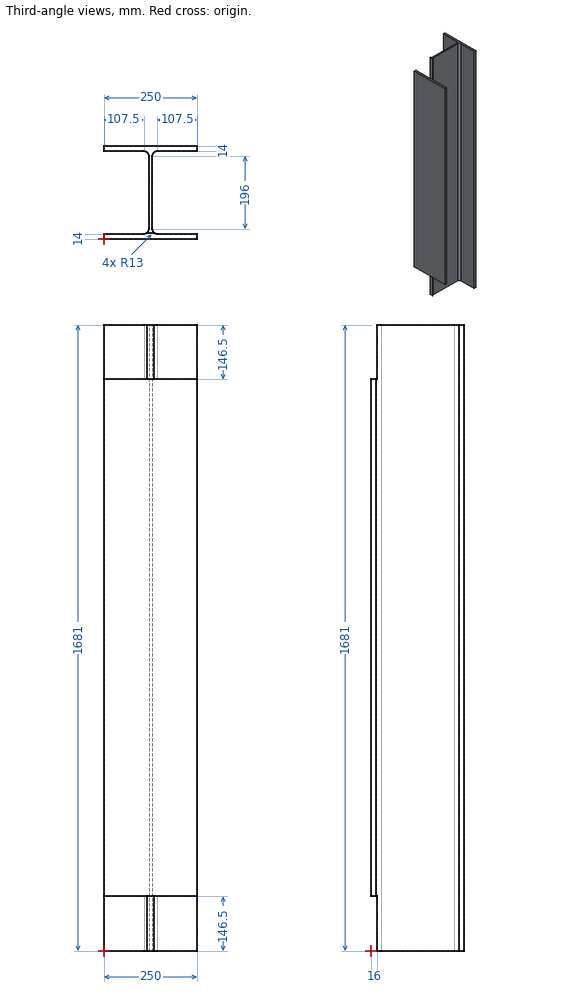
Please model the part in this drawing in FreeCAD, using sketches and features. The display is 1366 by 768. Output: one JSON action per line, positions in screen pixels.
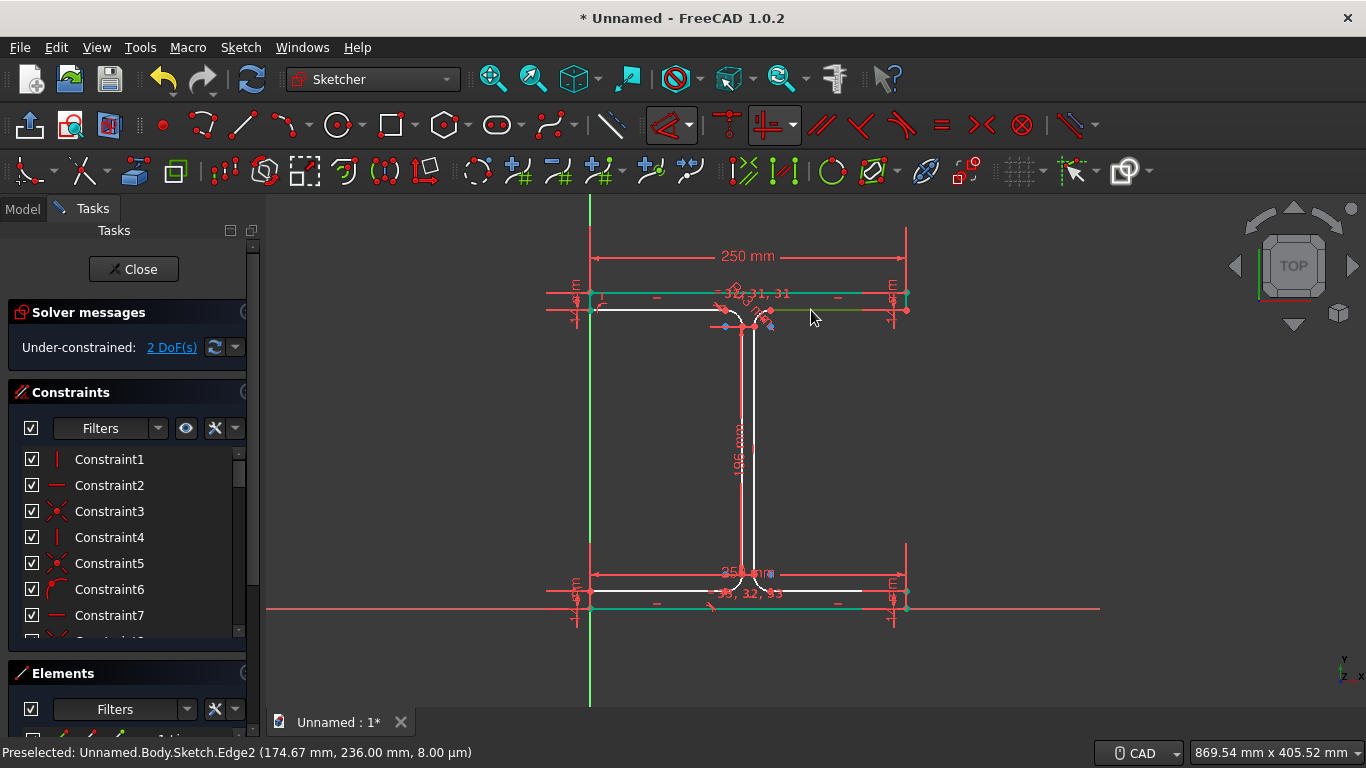
{"action": "left_click", "coordinate": [692, 126]}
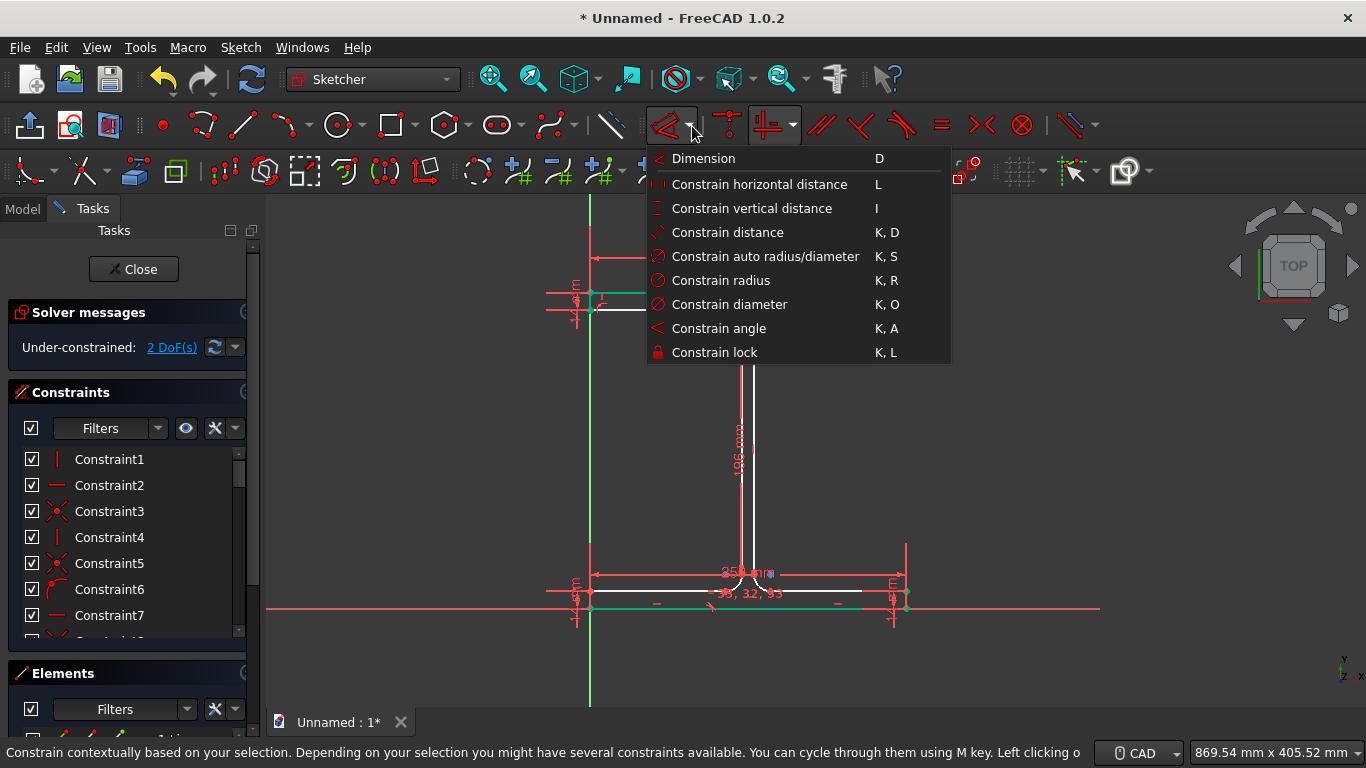
{"action": "left_click", "coordinate": [799, 184]}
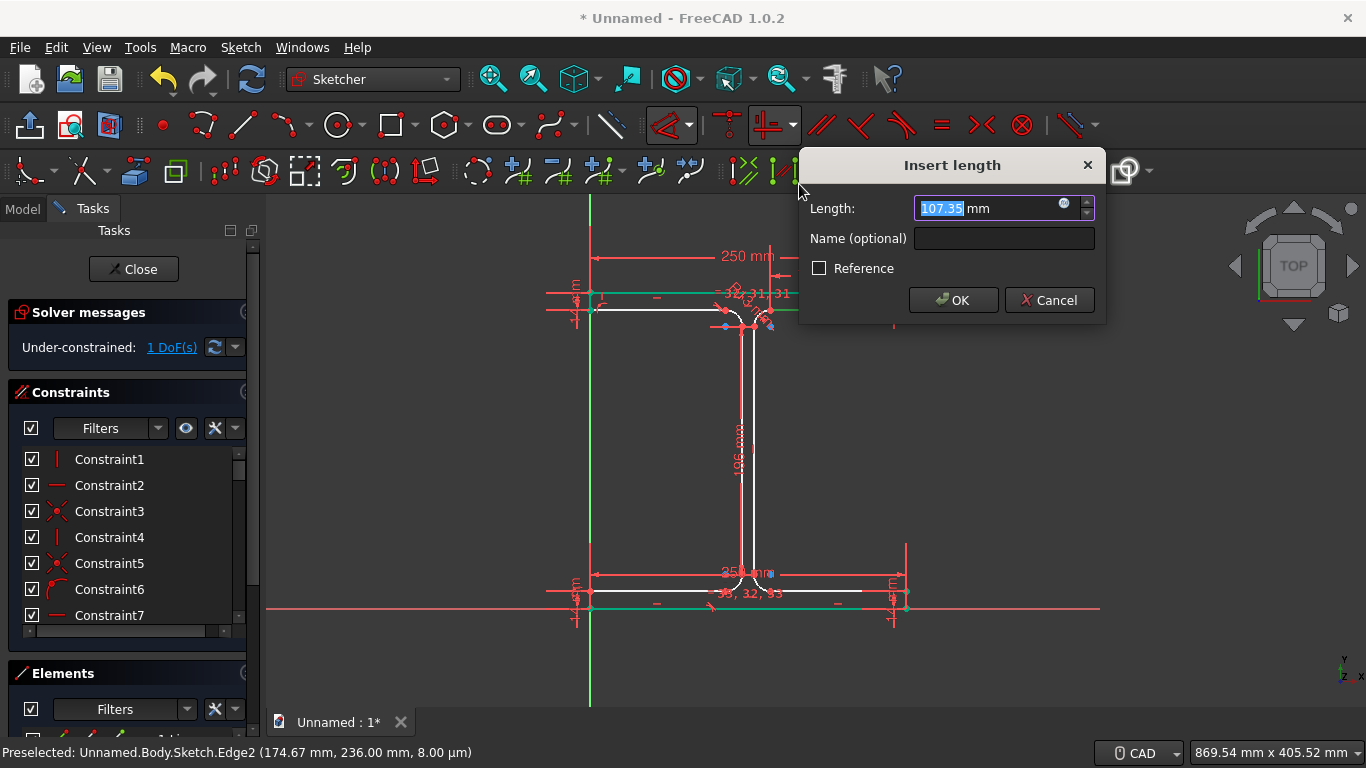
{"action": "type", "text": "107.5"}
{"action": "key", "text": "Return"}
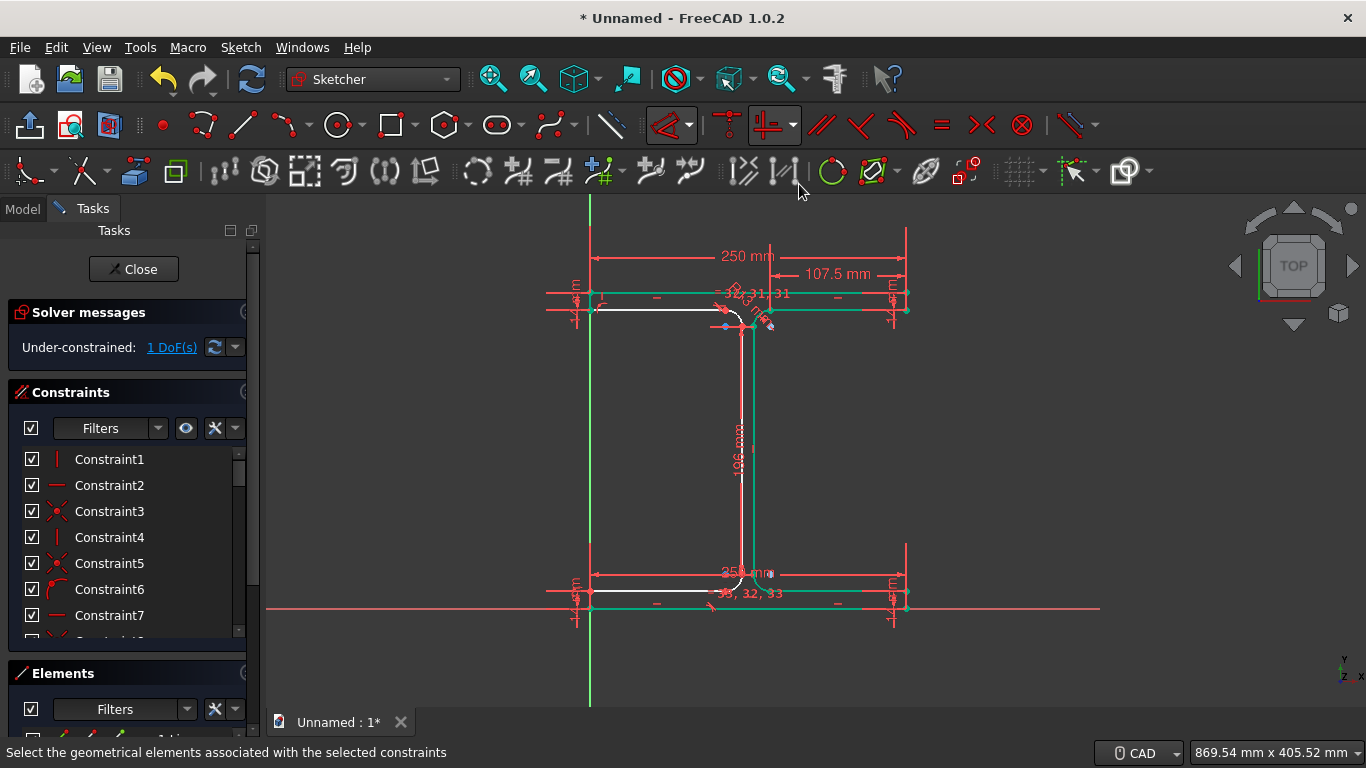
{"action": "left_click", "coordinate": [631, 310]}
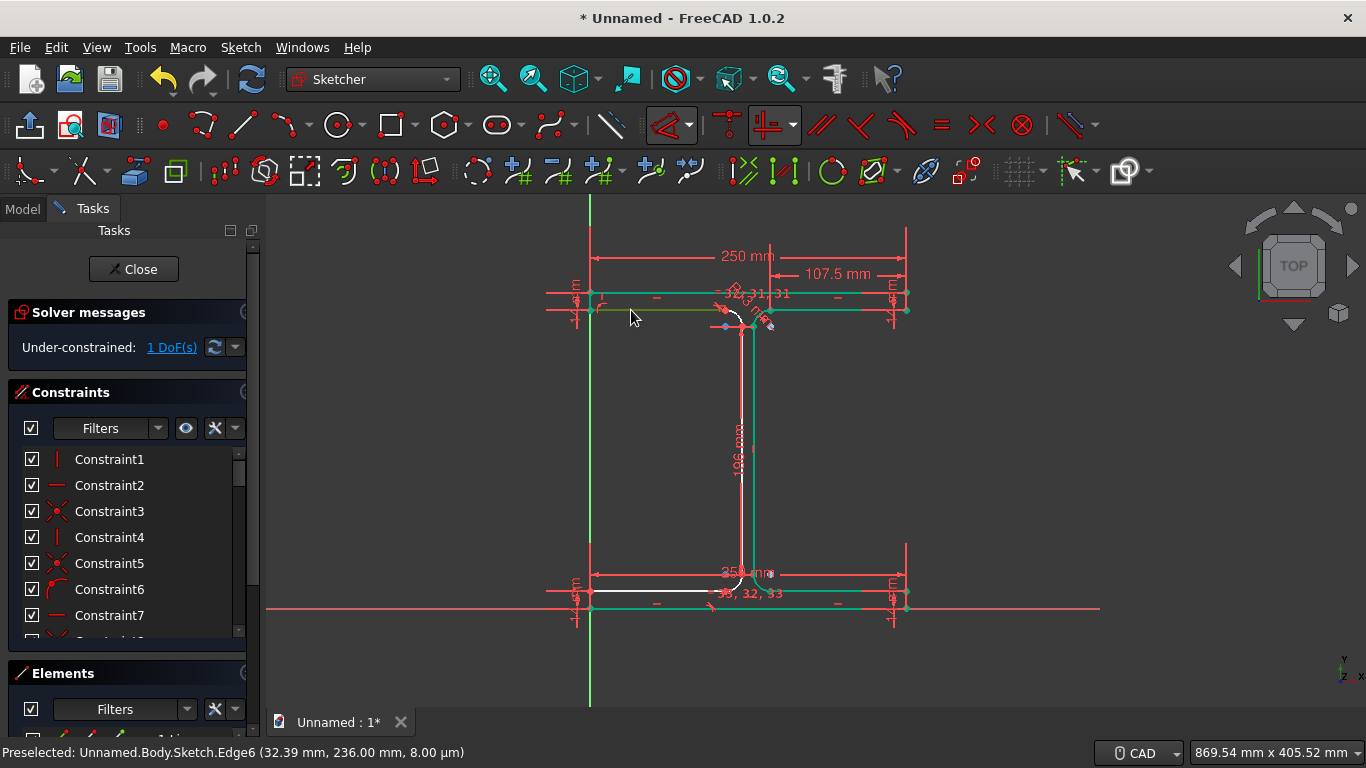
{"action": "left_click", "coordinate": [692, 126]}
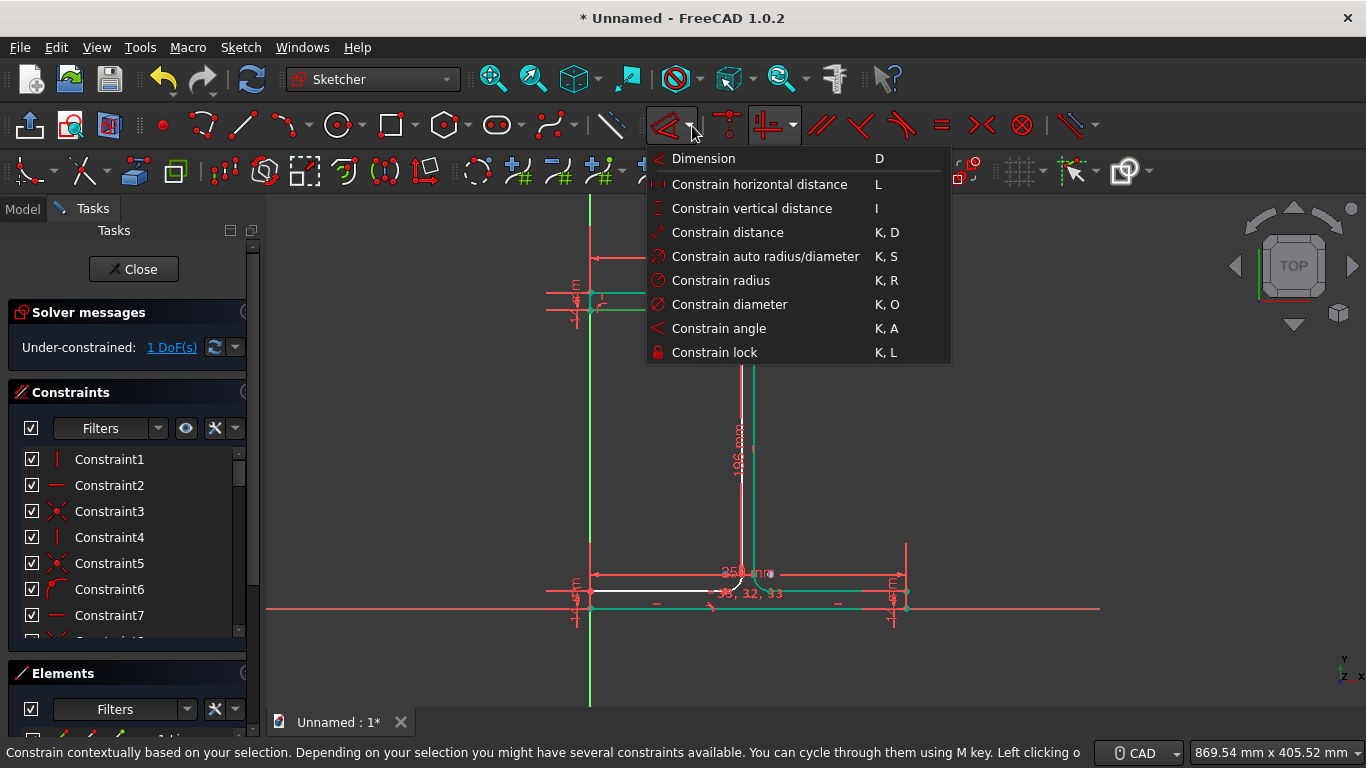
{"action": "left_click", "coordinate": [799, 184]}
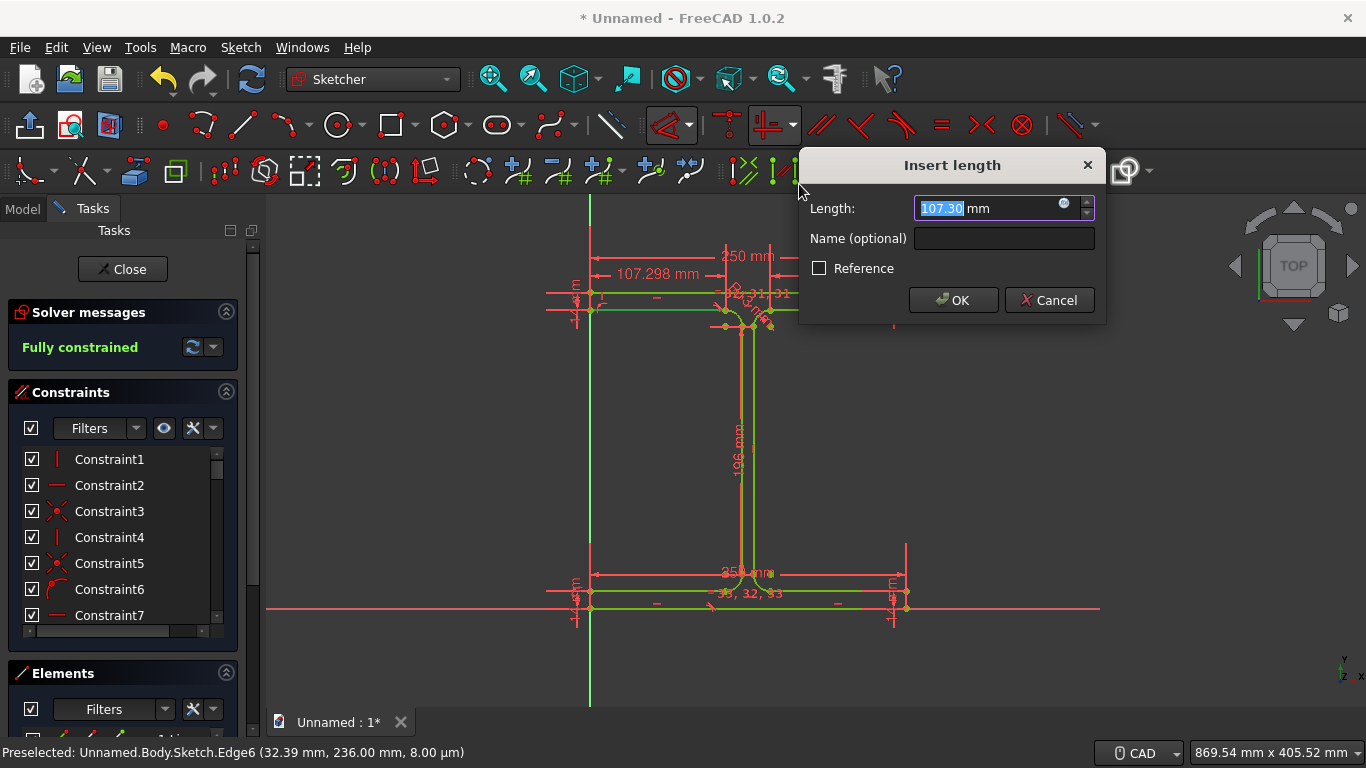
{"action": "type", "text": "107.5"}
{"action": "key", "text": "Return"}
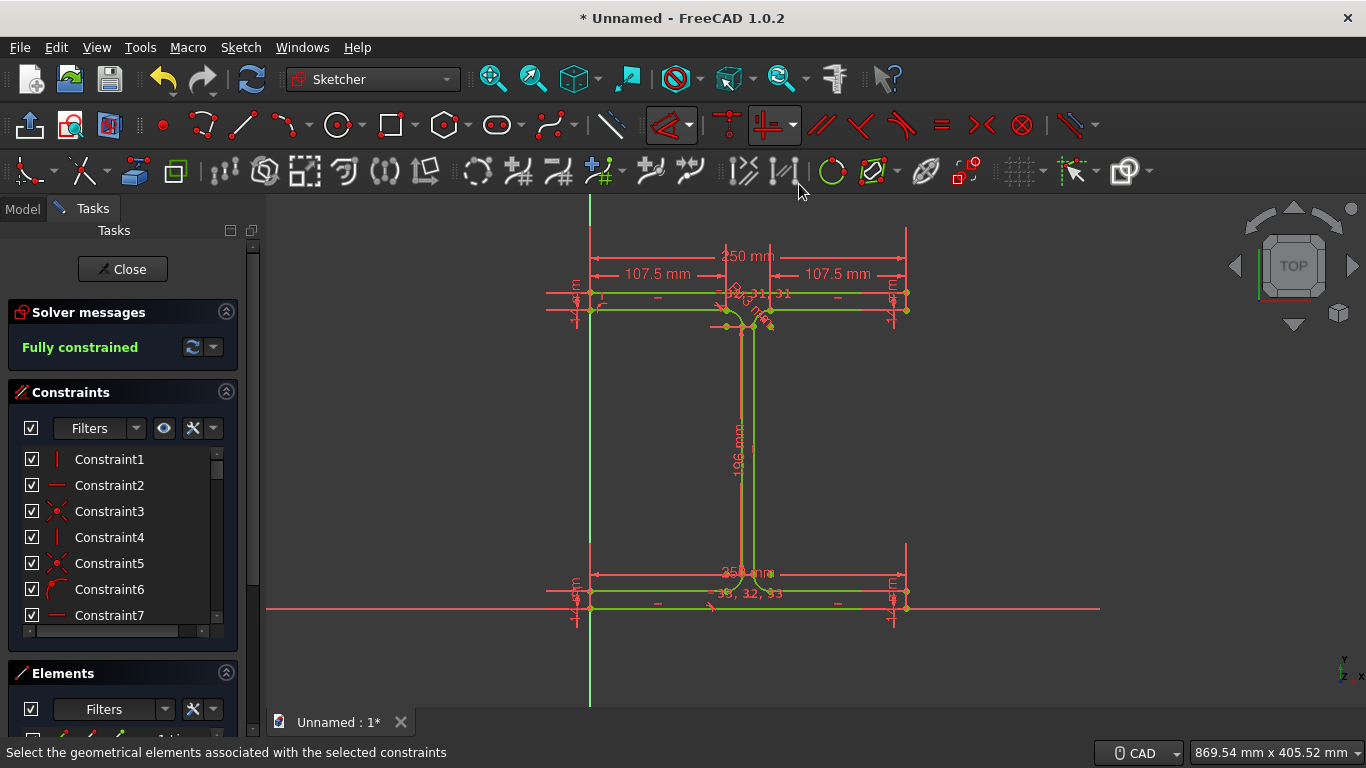
{"action": "left_click", "coordinate": [123, 269]}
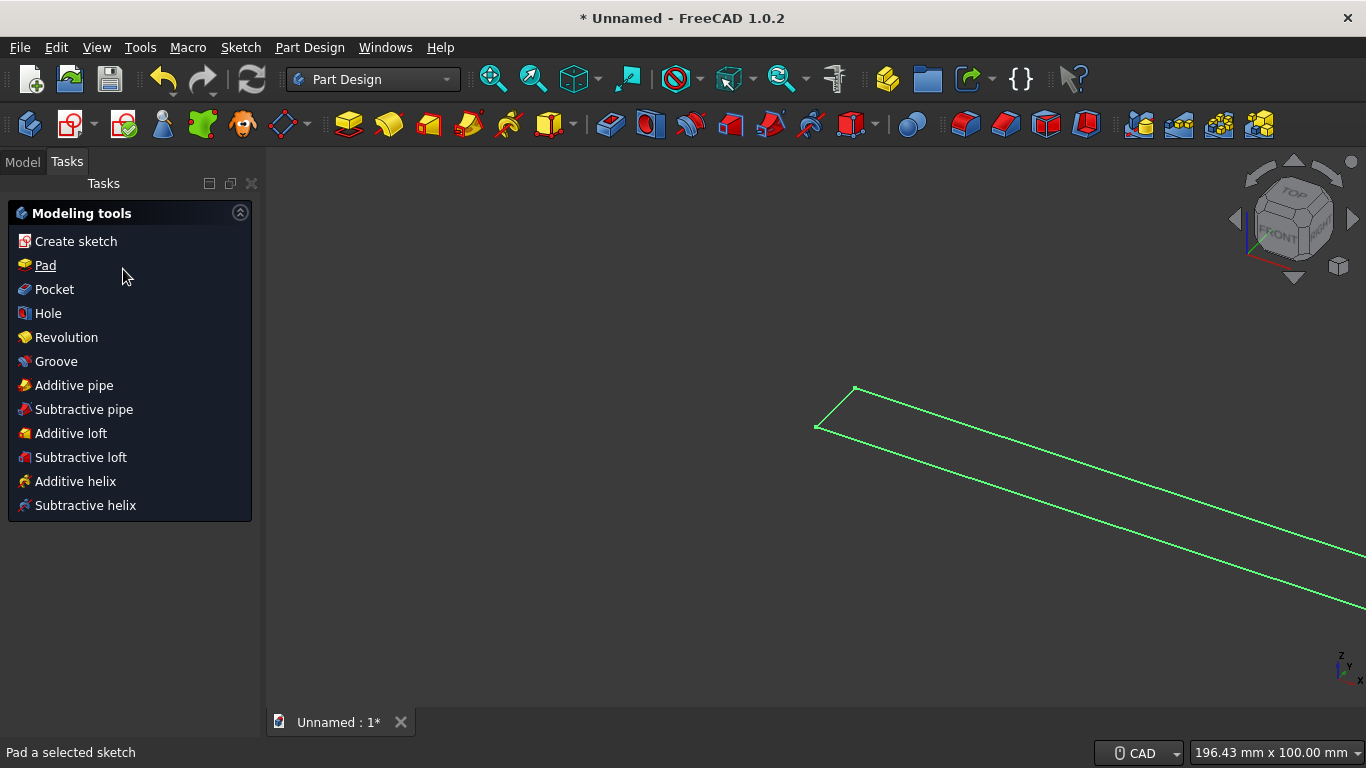
{"action": "left_click", "coordinate": [350, 124]}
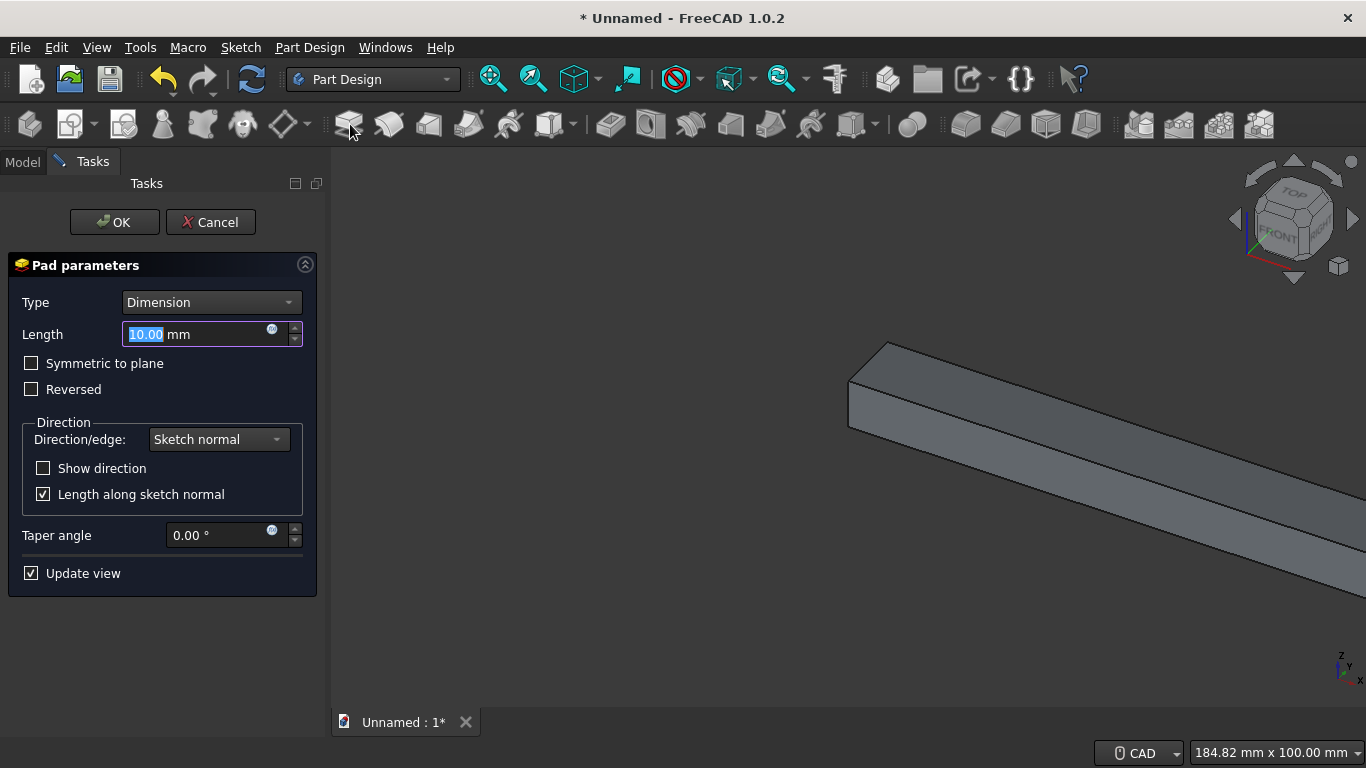
{"action": "type", "text": "1681"}
{"action": "key", "text": "Tab"}